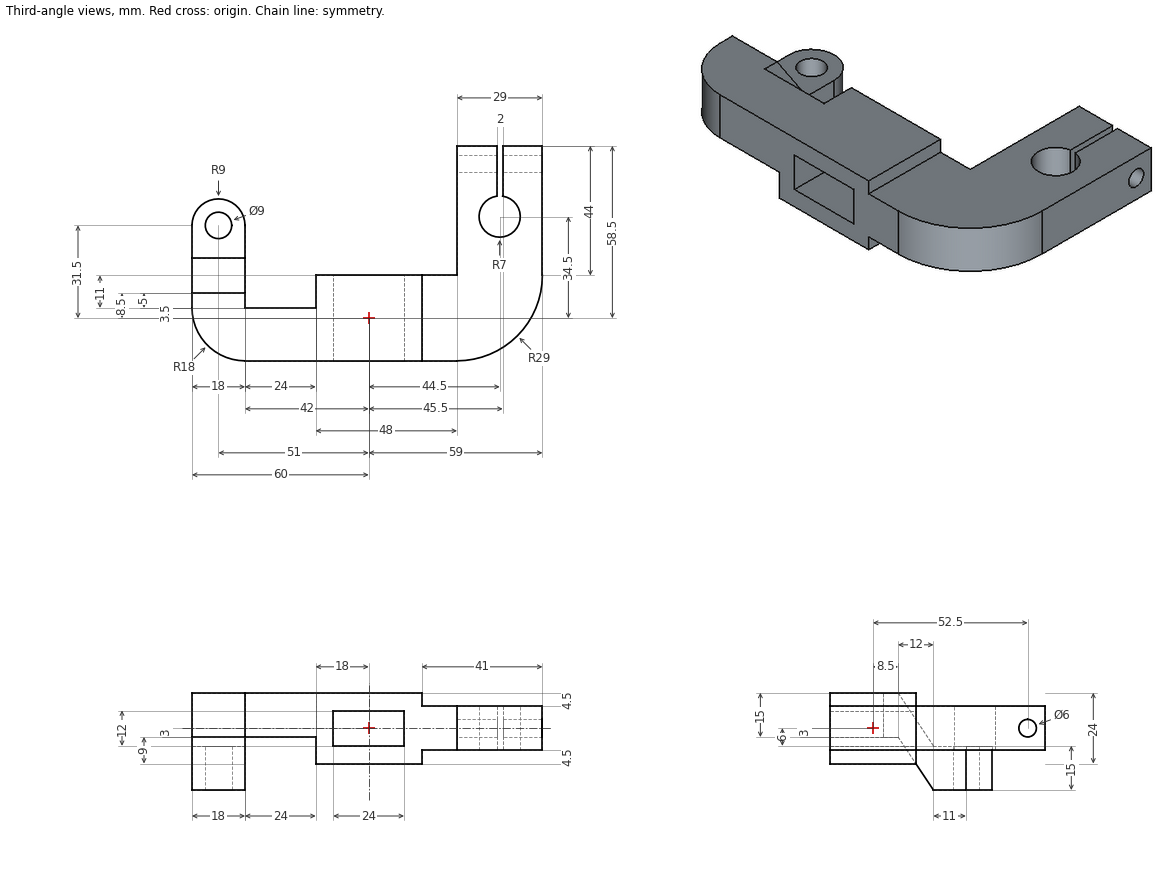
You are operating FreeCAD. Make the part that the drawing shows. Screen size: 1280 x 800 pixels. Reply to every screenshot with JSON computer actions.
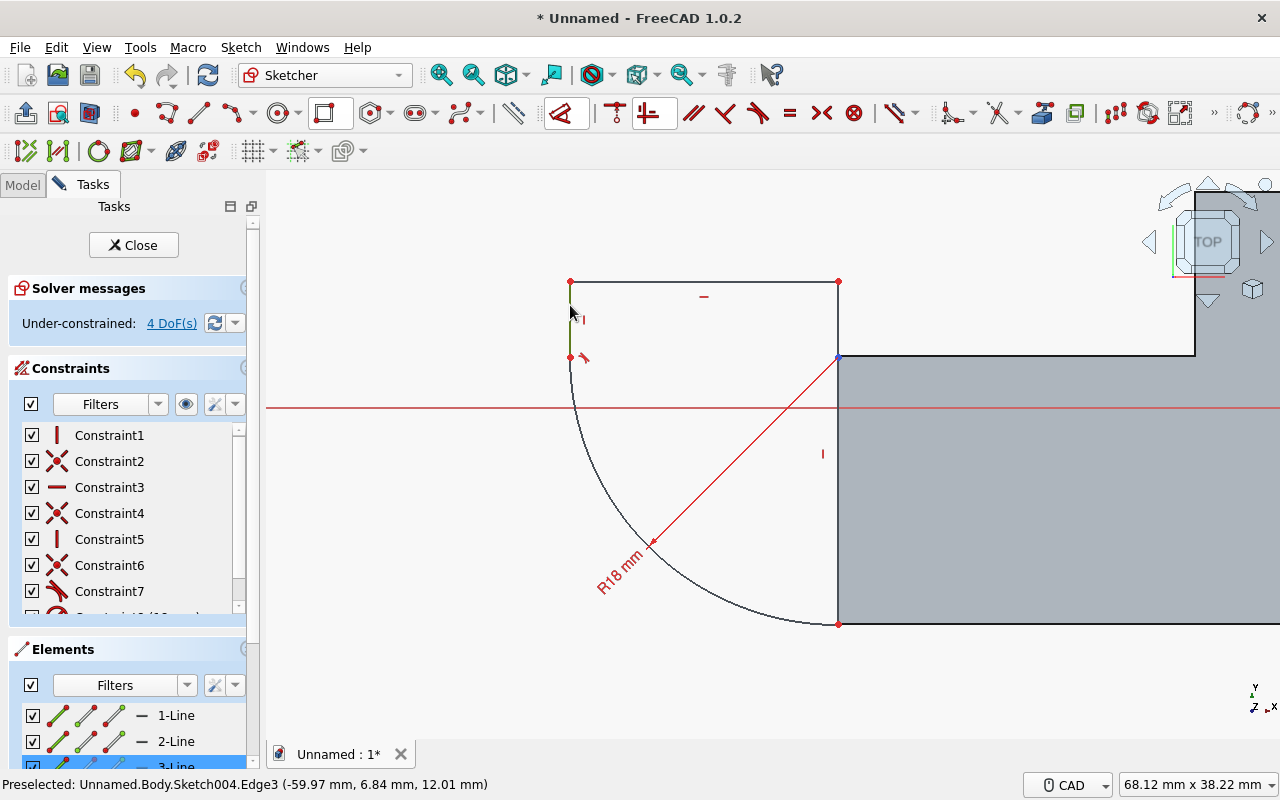
{"action": "key", "text": "i"}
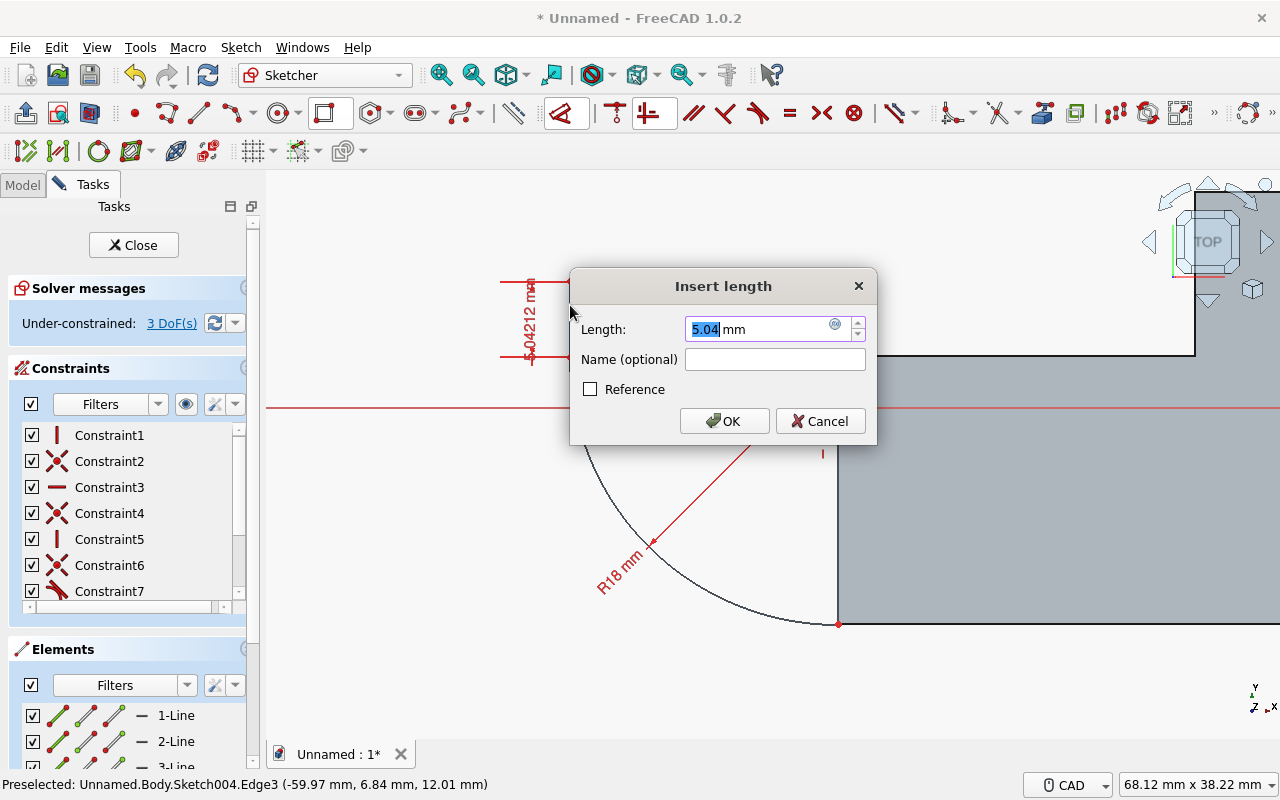
{"action": "type", "text": "5"}
{"action": "key", "text": "Return"}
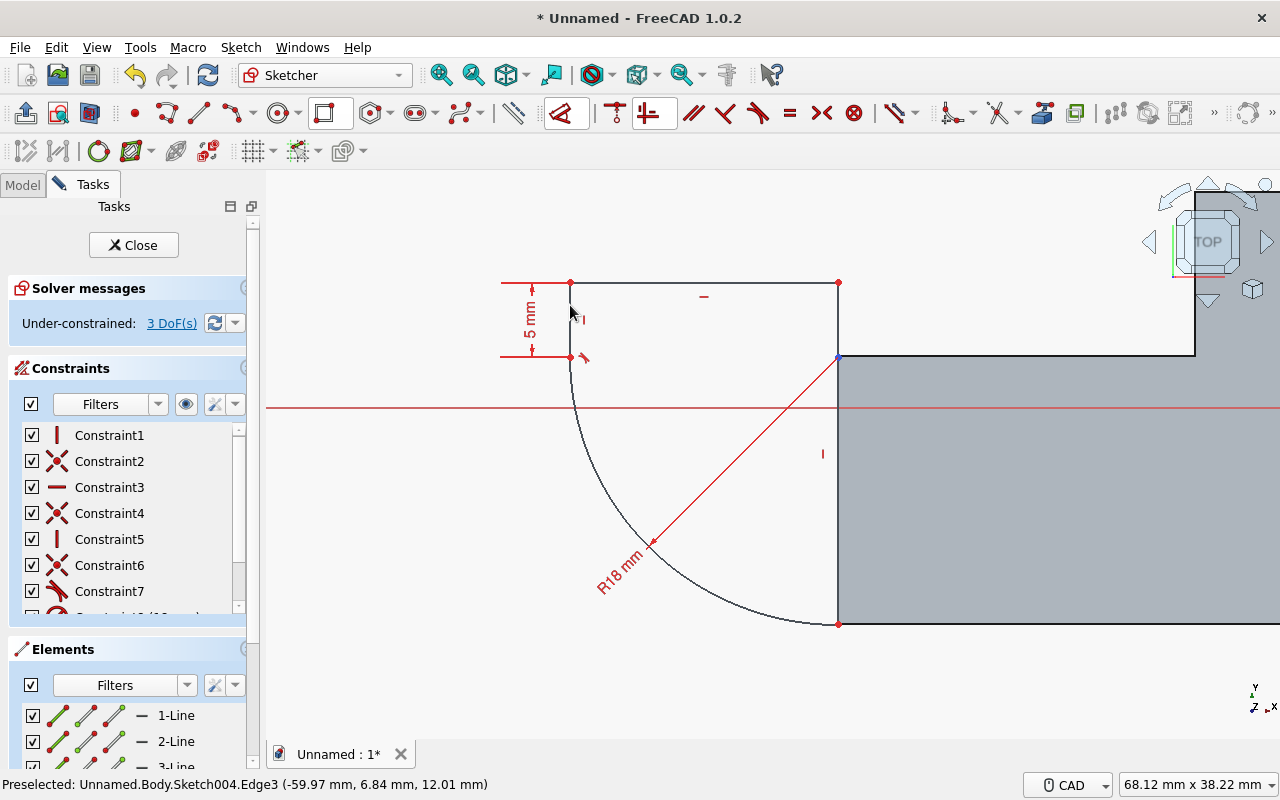
{"action": "left_click", "coordinate": [758, 283]}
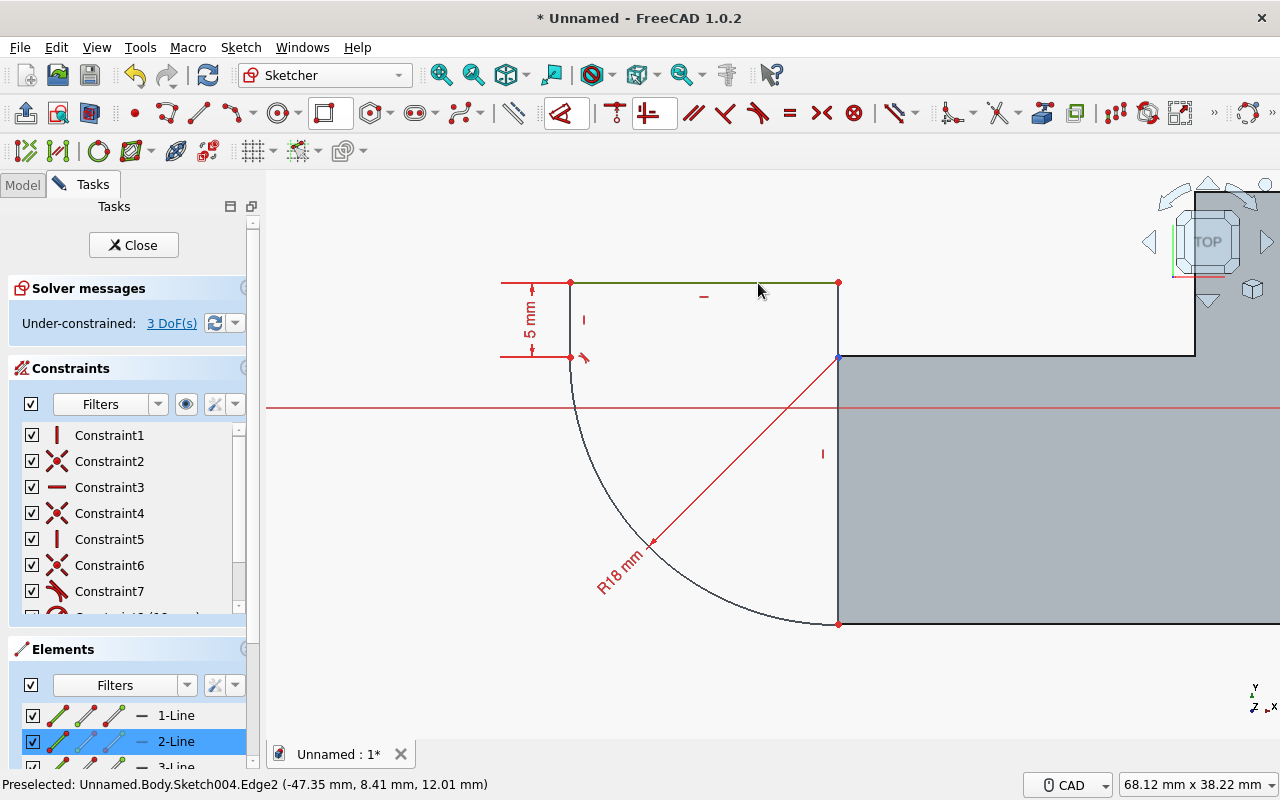
{"action": "left_click", "coordinate": [584, 114]}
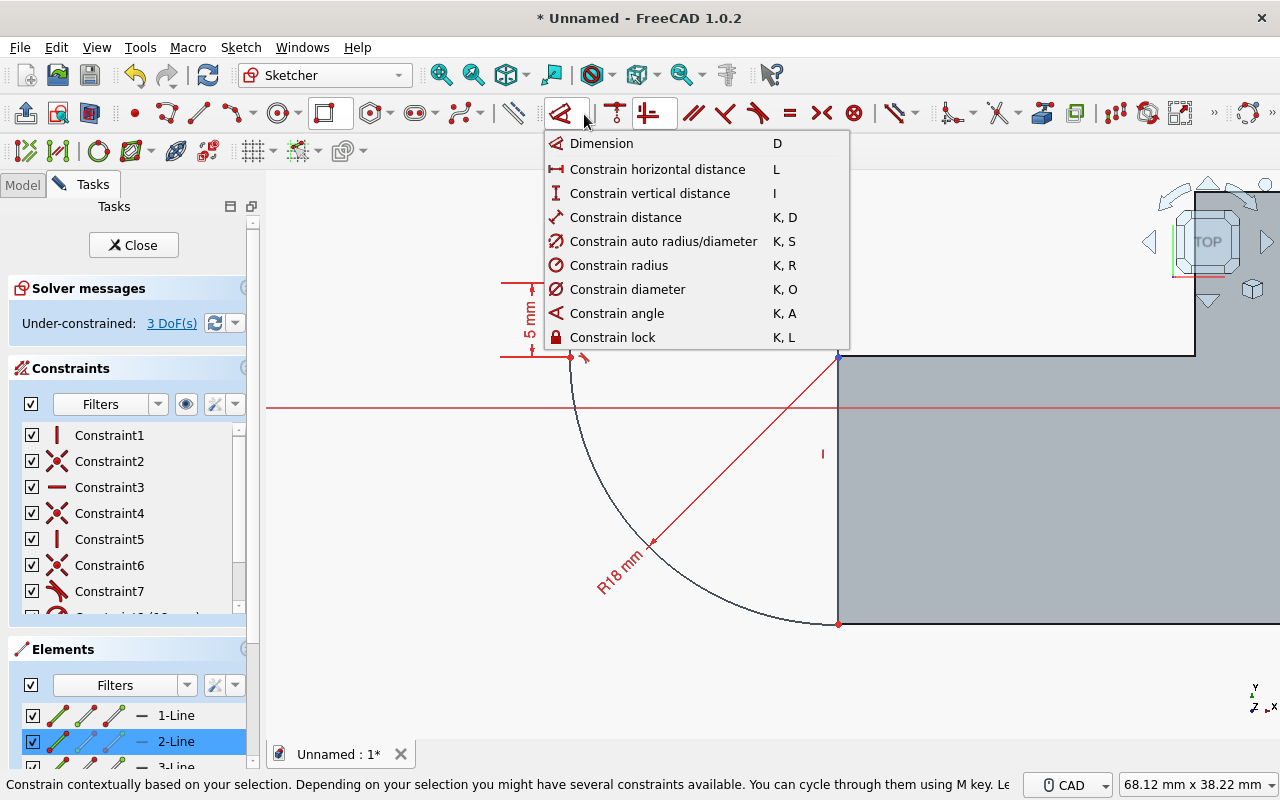
{"action": "left_click", "coordinate": [697, 169]}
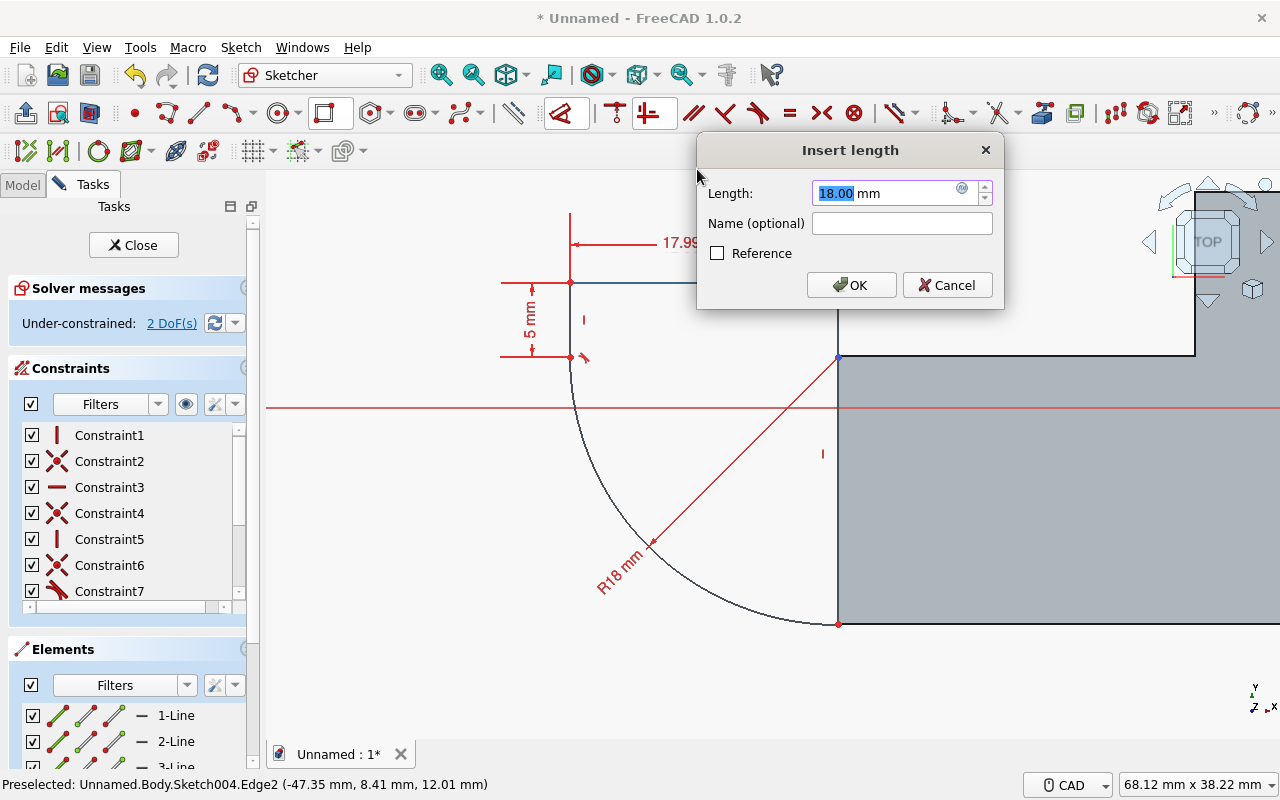
{"action": "type", "text": "18"}
{"action": "key", "text": "Return"}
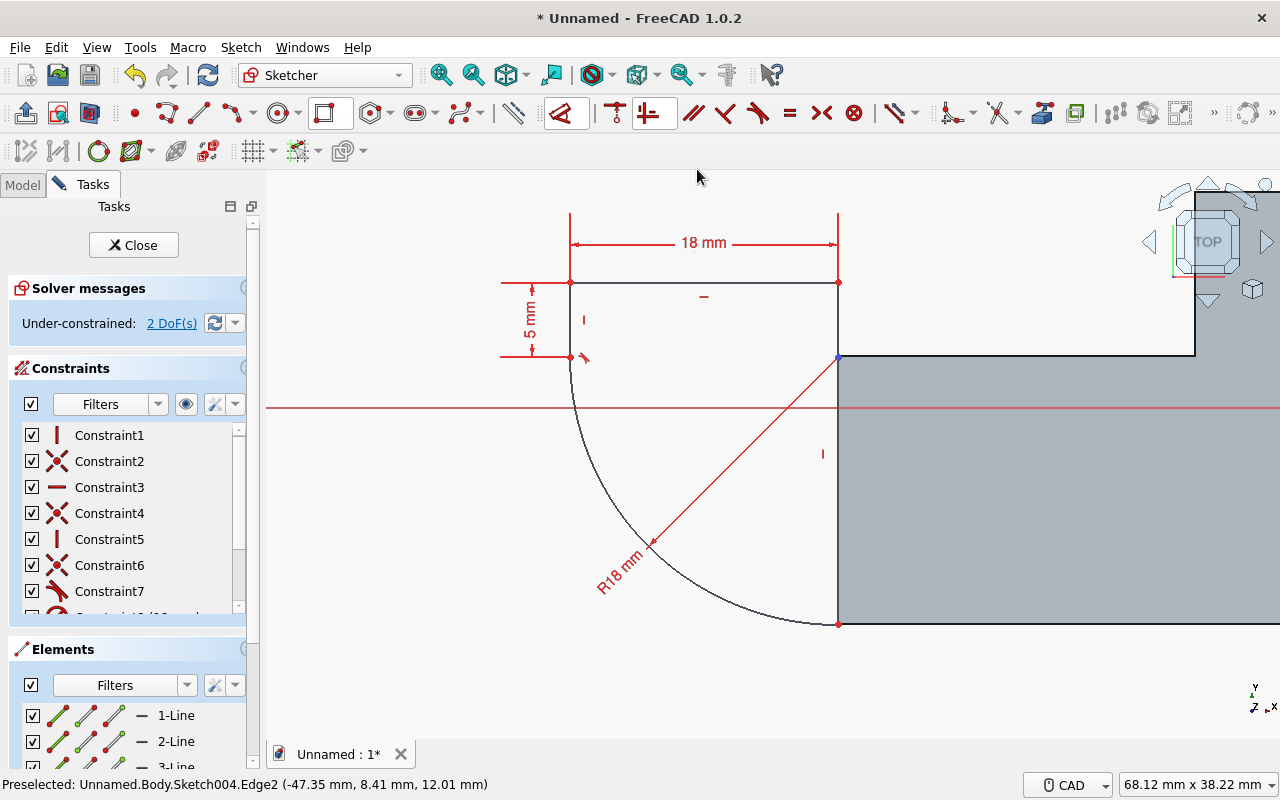
{"action": "left_click", "coordinate": [838, 625]}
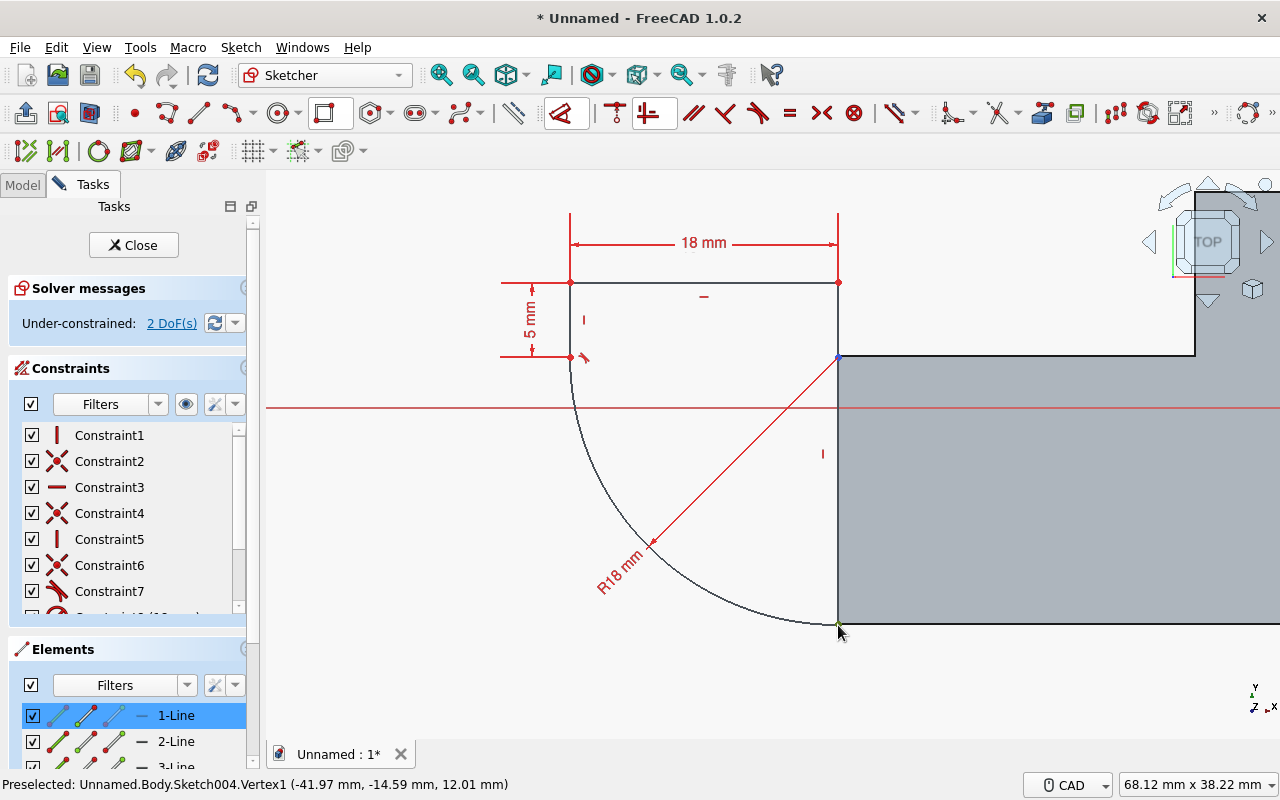
{"action": "key", "text": "l"}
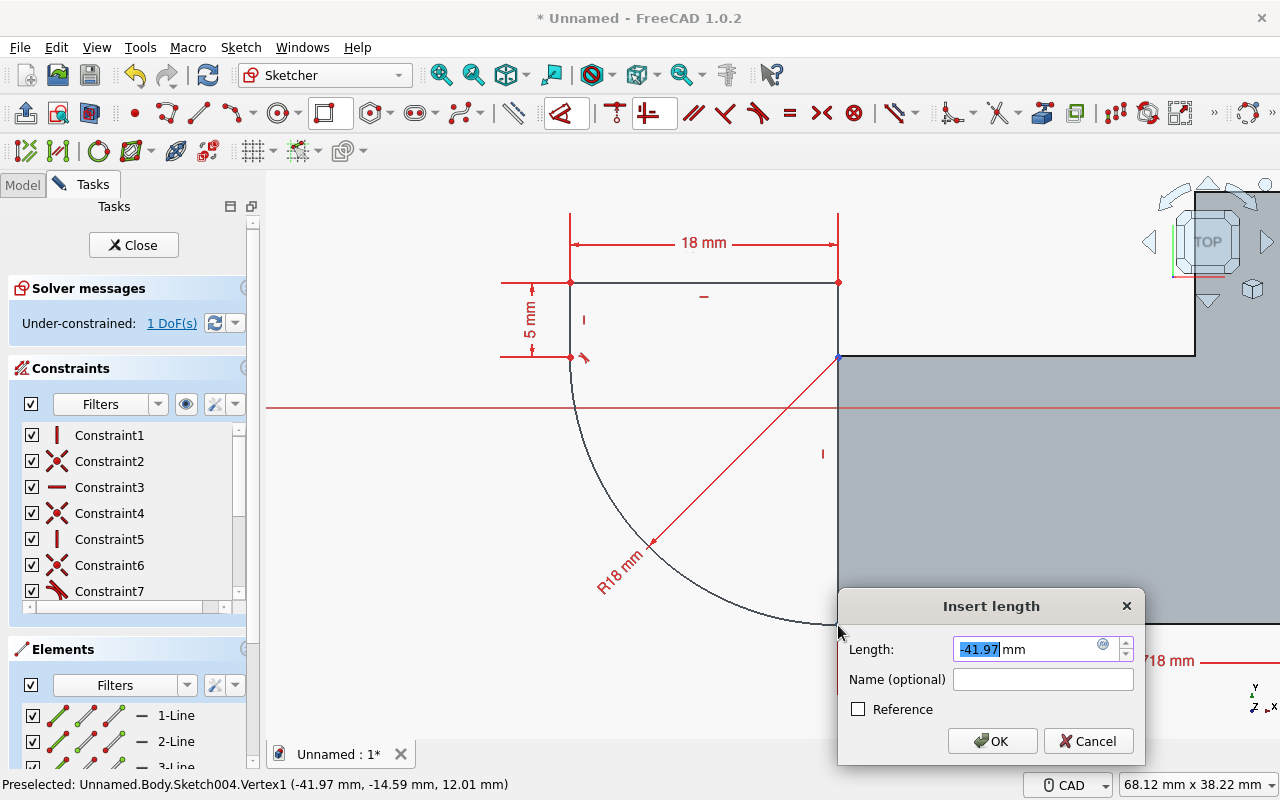
{"action": "type", "text": "-42"}
{"action": "key", "text": "Return"}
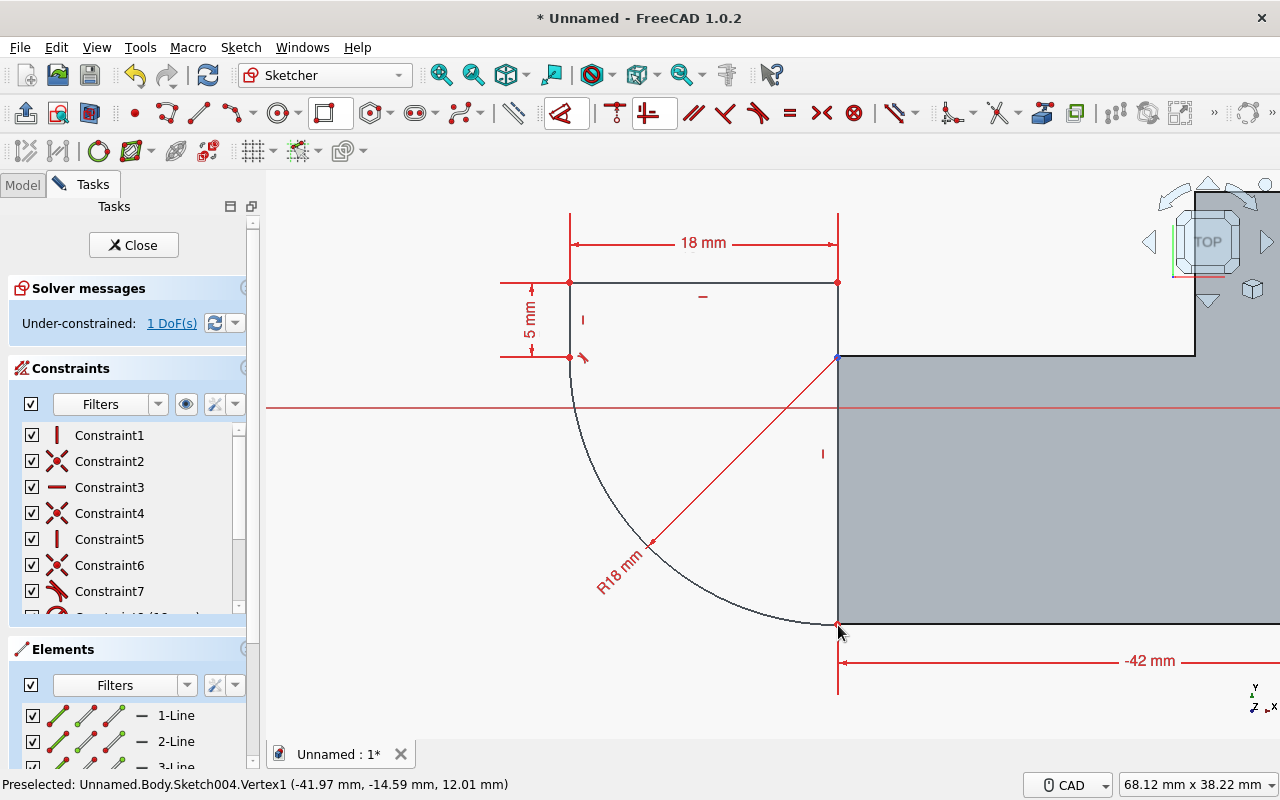
{"action": "left_click", "coordinate": [838, 283]}